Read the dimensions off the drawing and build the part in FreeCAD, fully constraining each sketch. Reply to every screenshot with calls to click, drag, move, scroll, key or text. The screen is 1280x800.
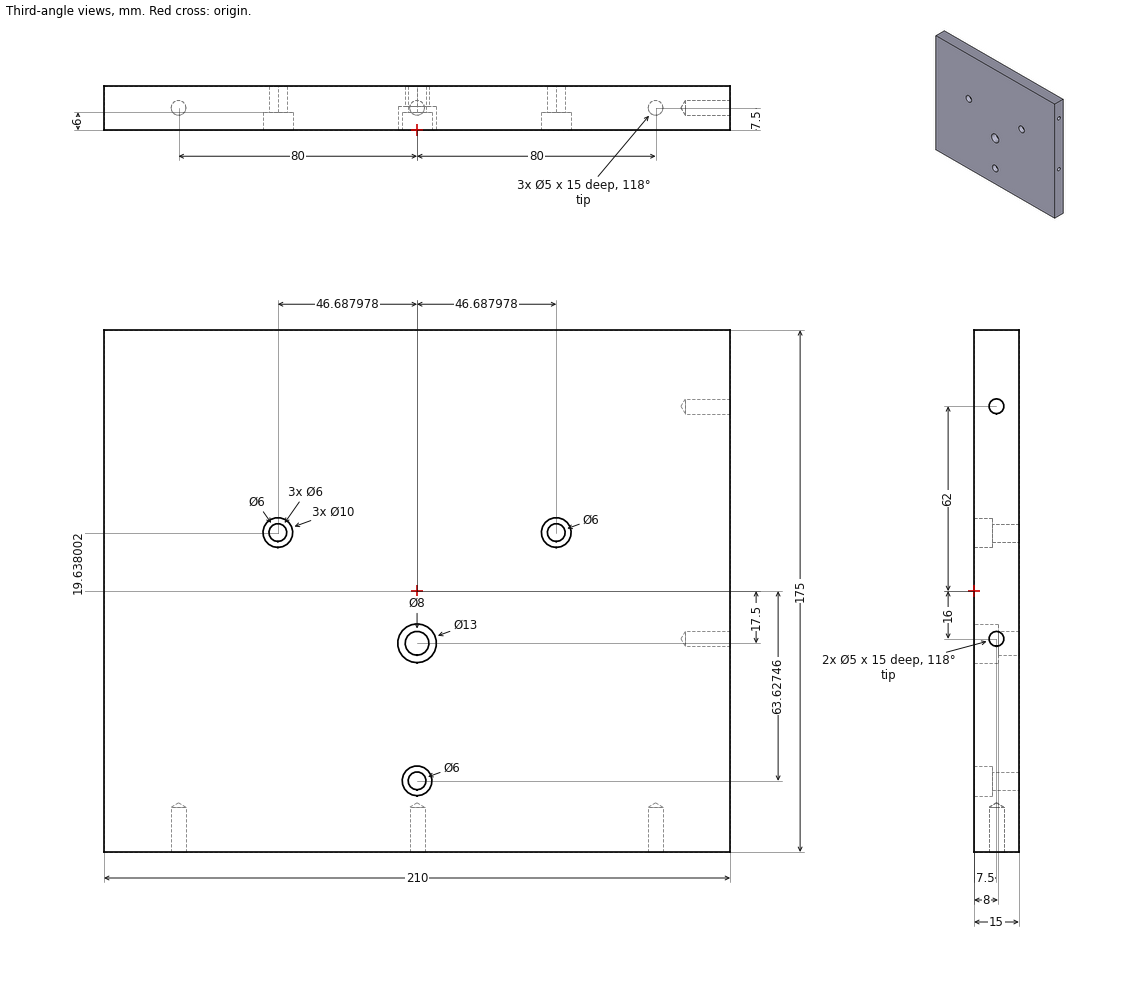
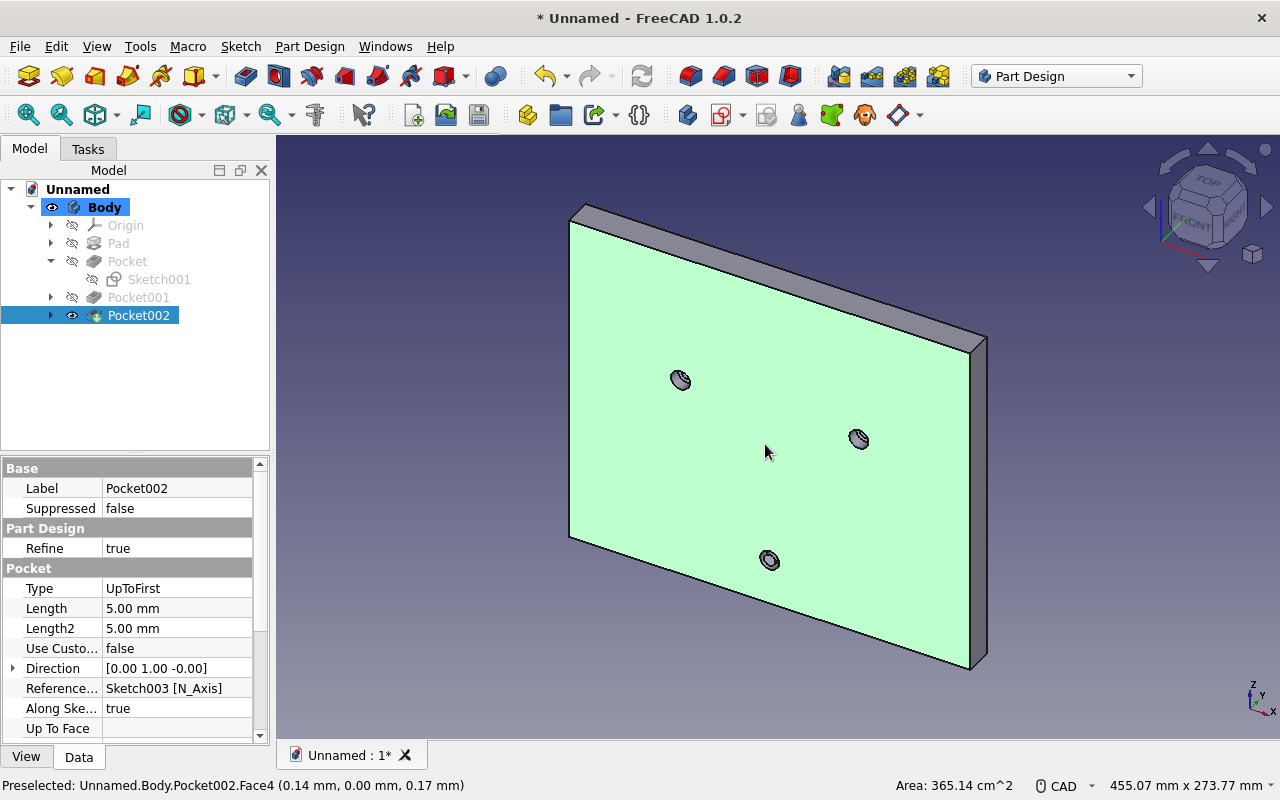
click(720, 116)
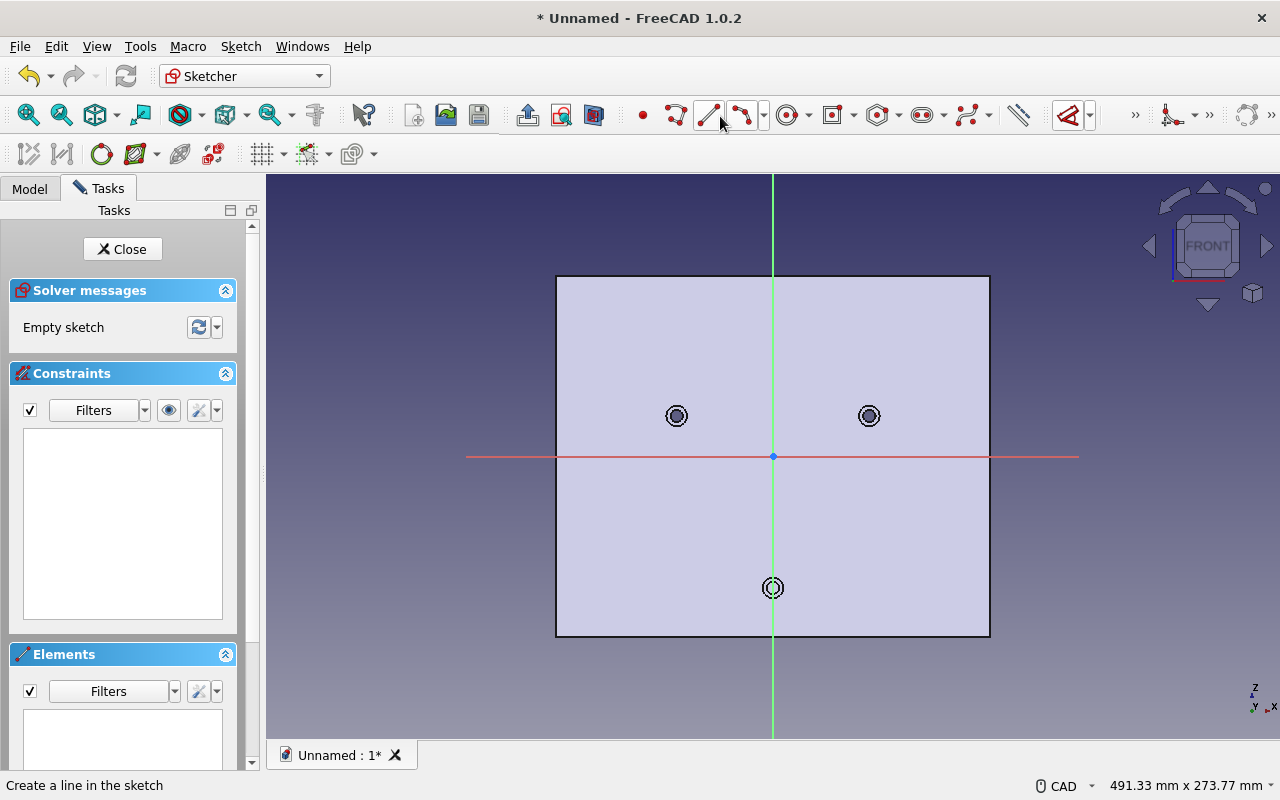
scroll(777, 595, up, 15)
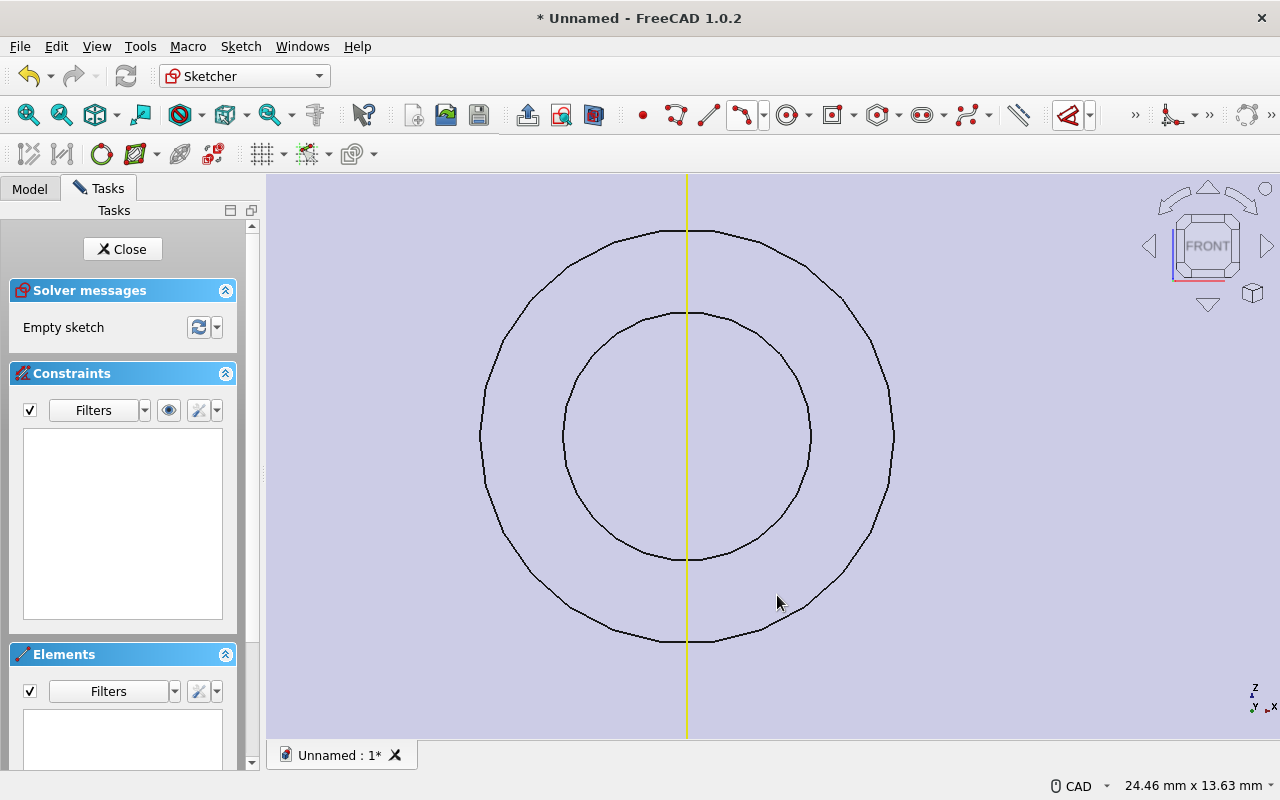
scroll(652, 396, up, 2)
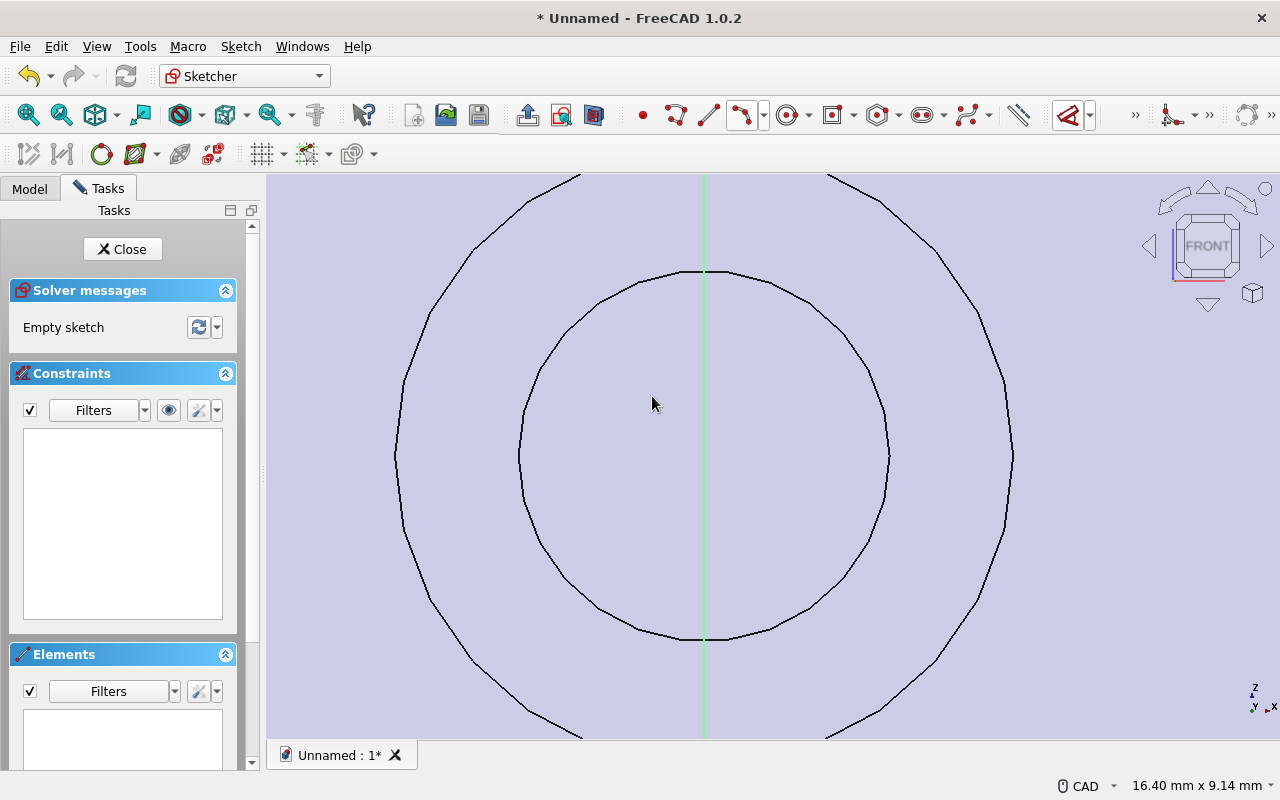
click(786, 116)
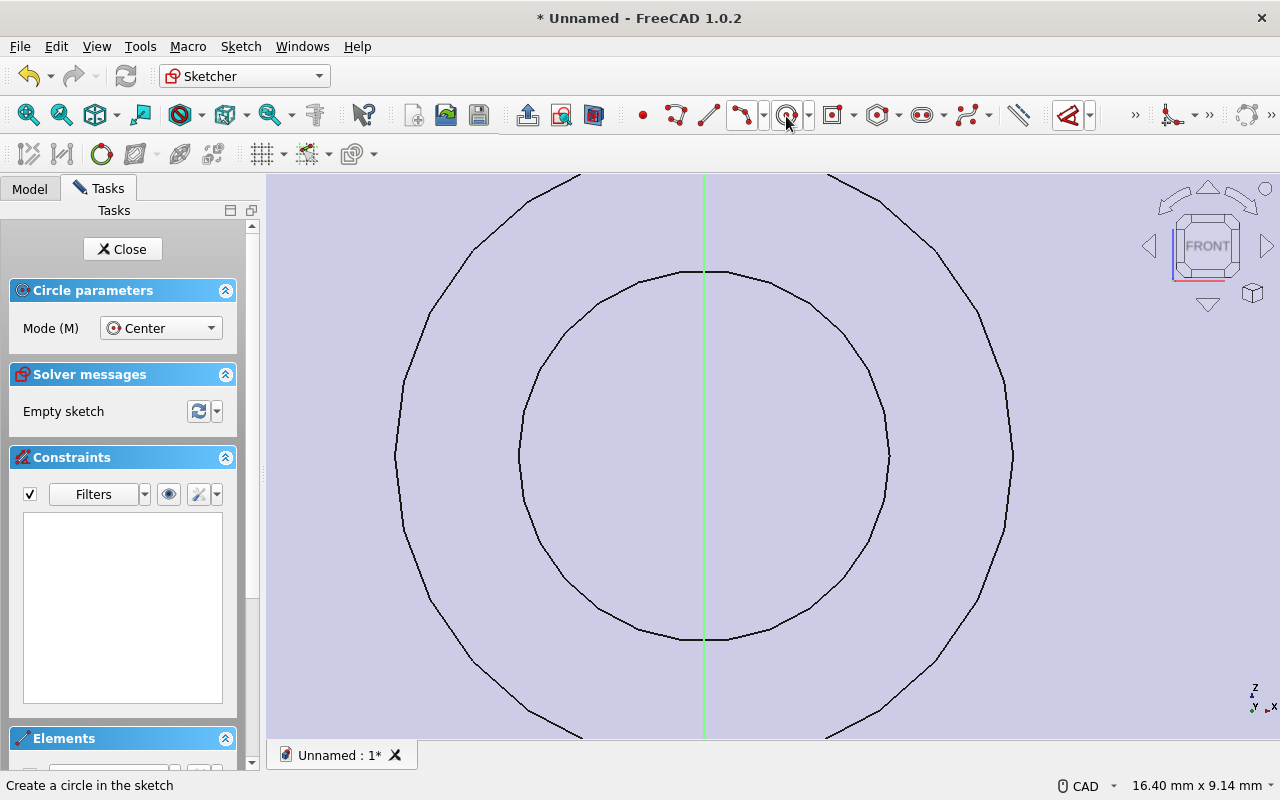
click(704, 456)
click(835, 325)
key(Escape)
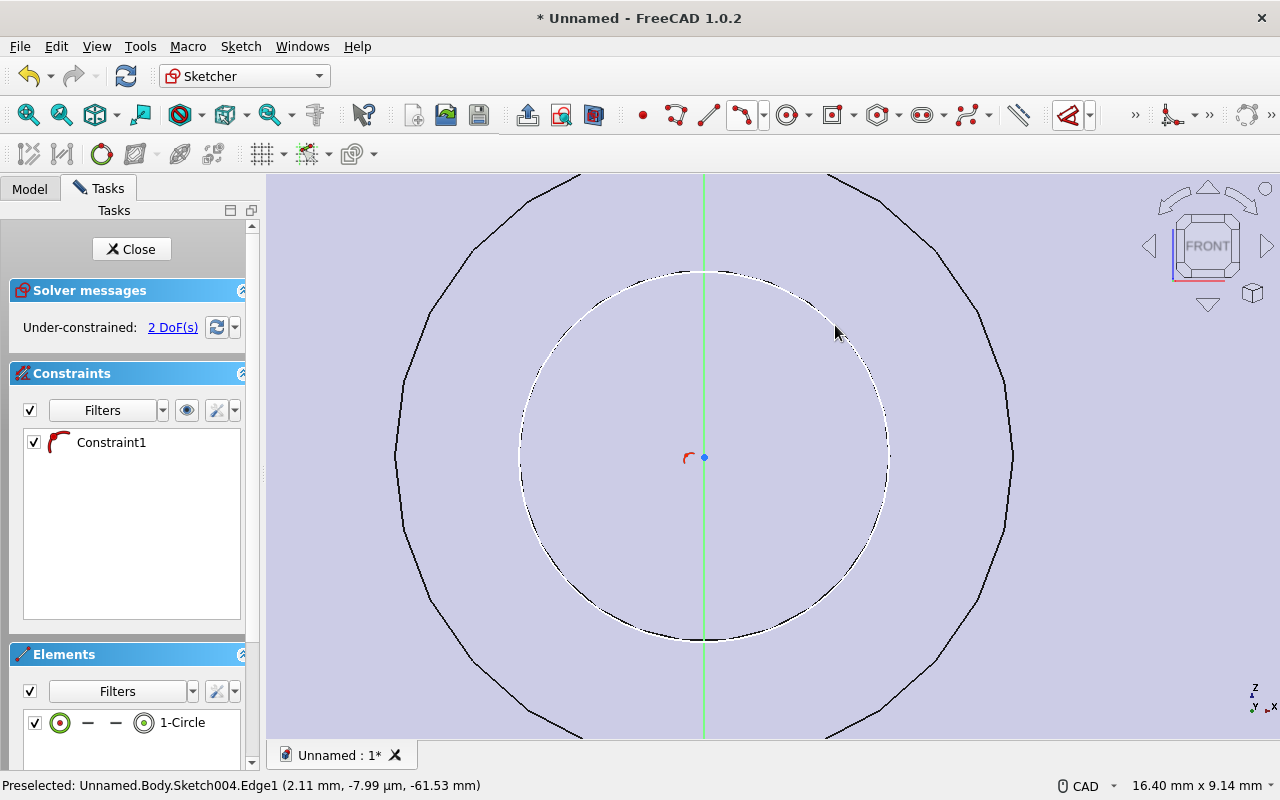
click(835, 326)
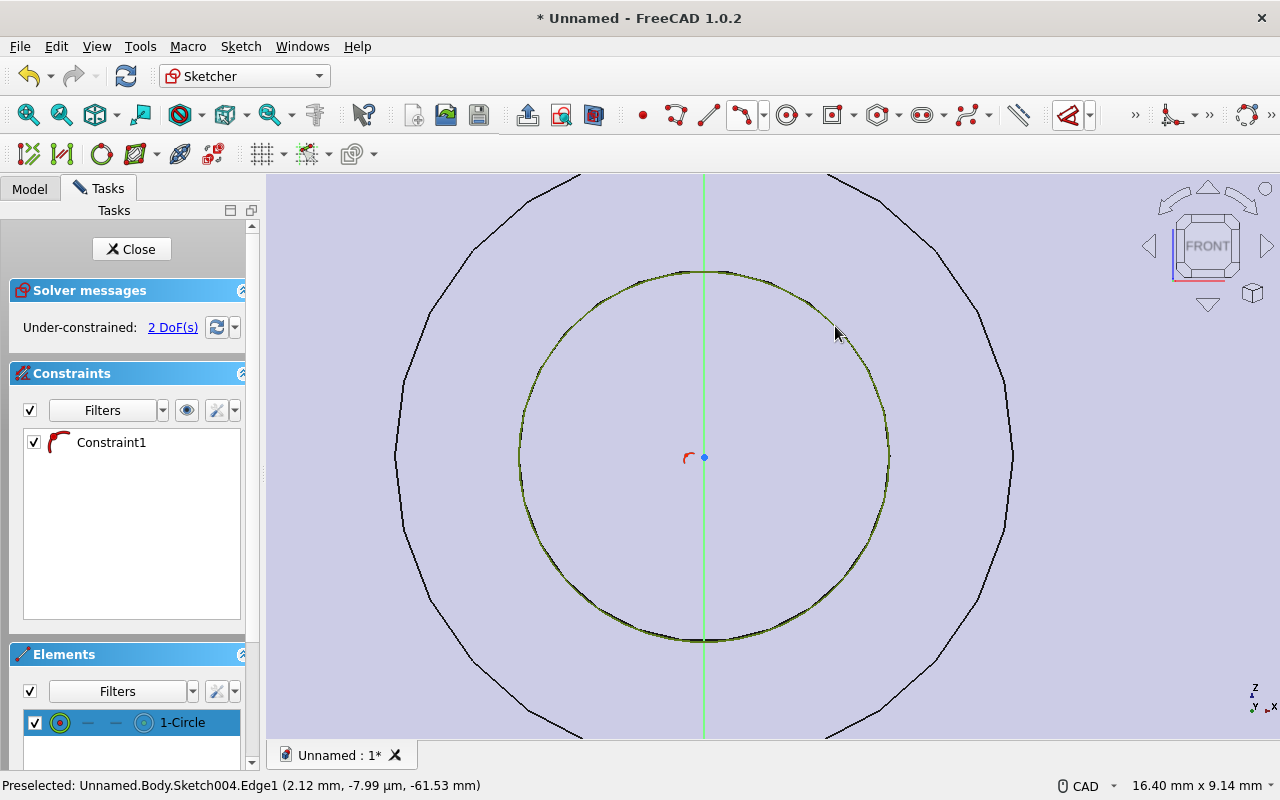
key(k)
key(o)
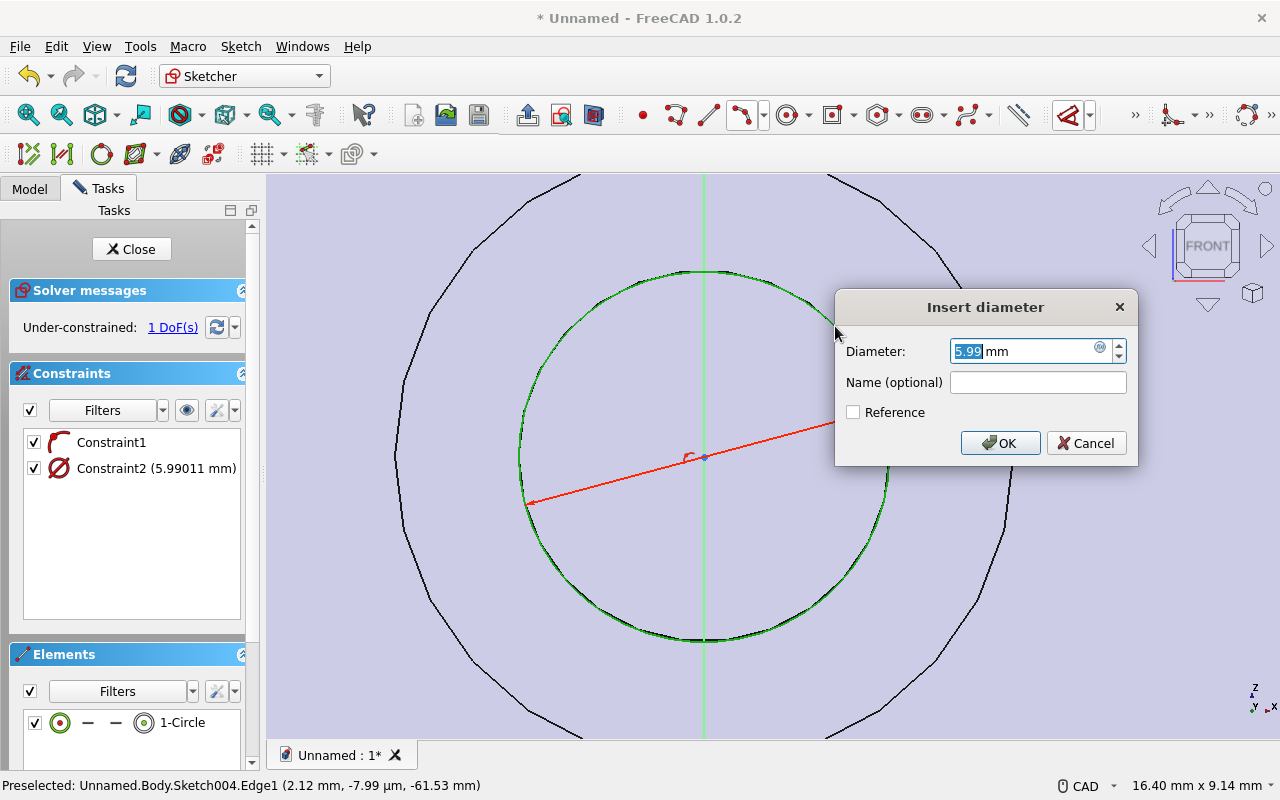
text(6)
key(Return)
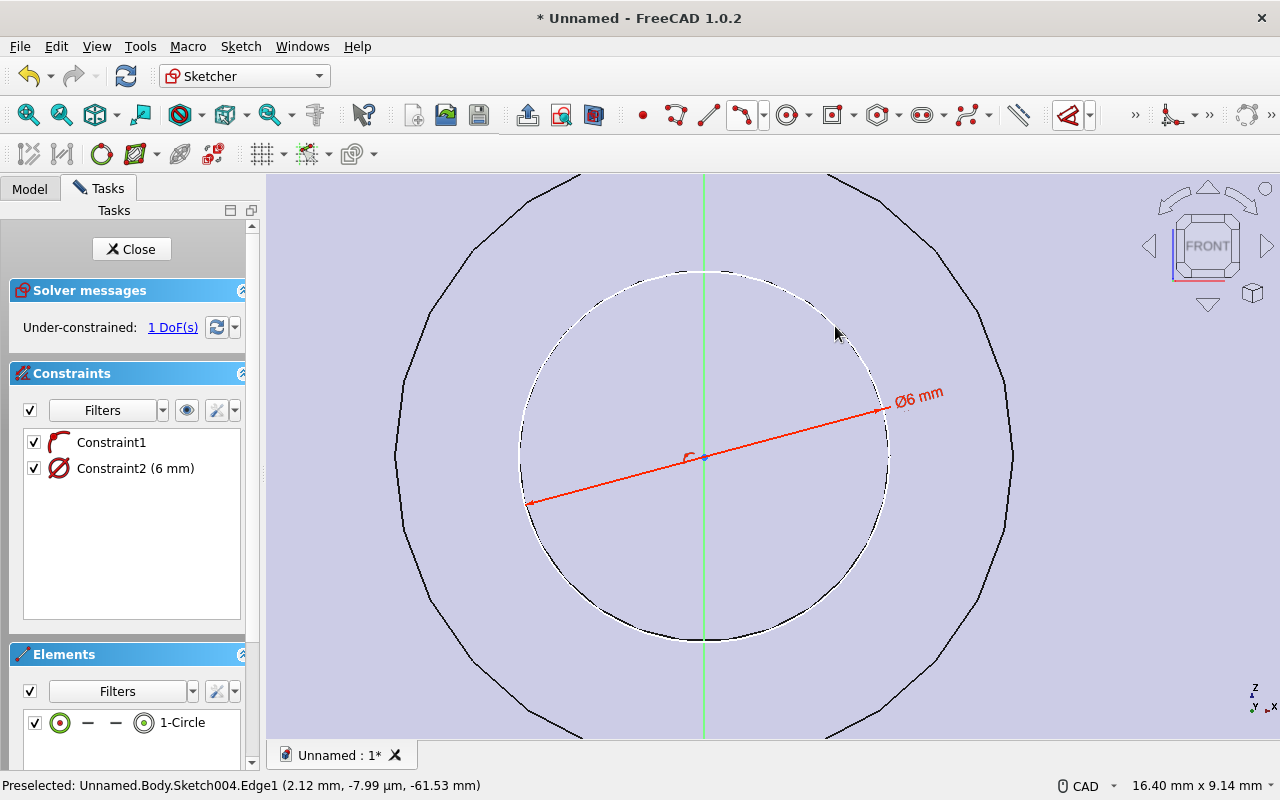
click(704, 457)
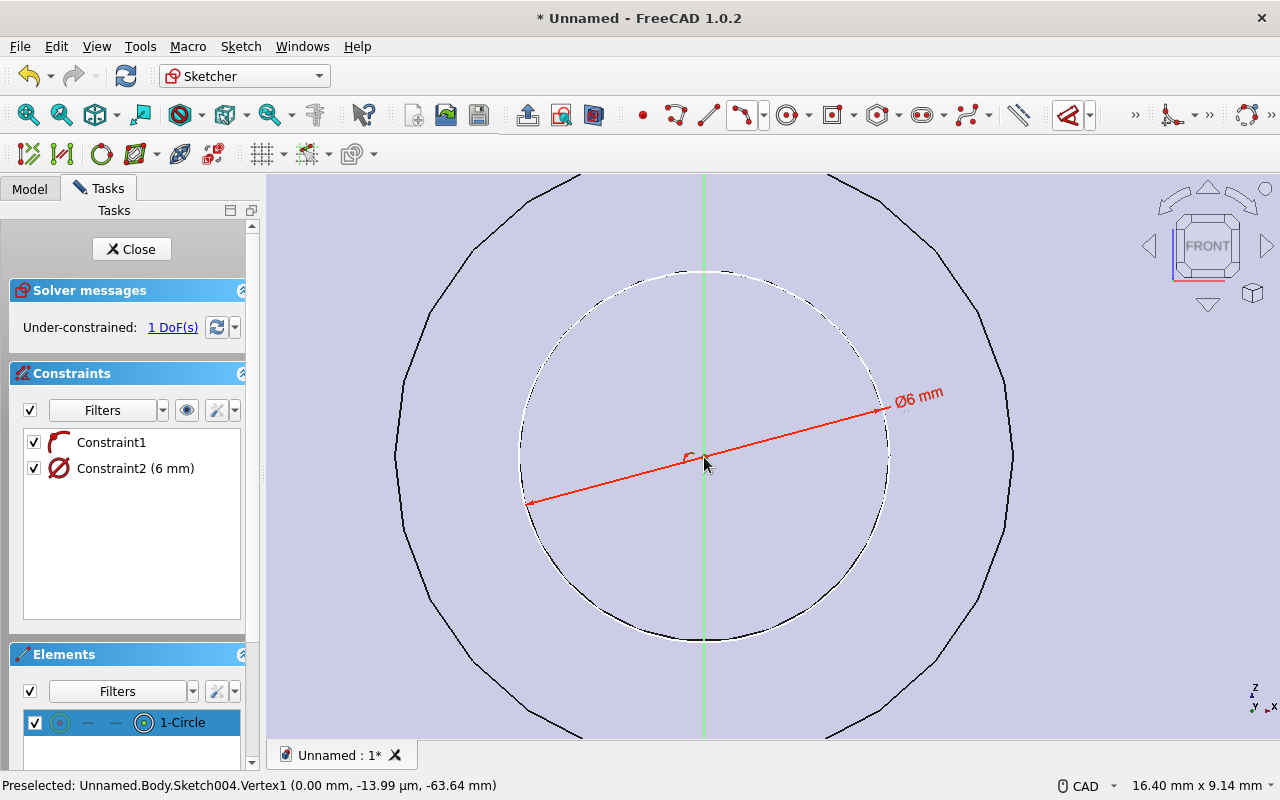
click(1090, 116)